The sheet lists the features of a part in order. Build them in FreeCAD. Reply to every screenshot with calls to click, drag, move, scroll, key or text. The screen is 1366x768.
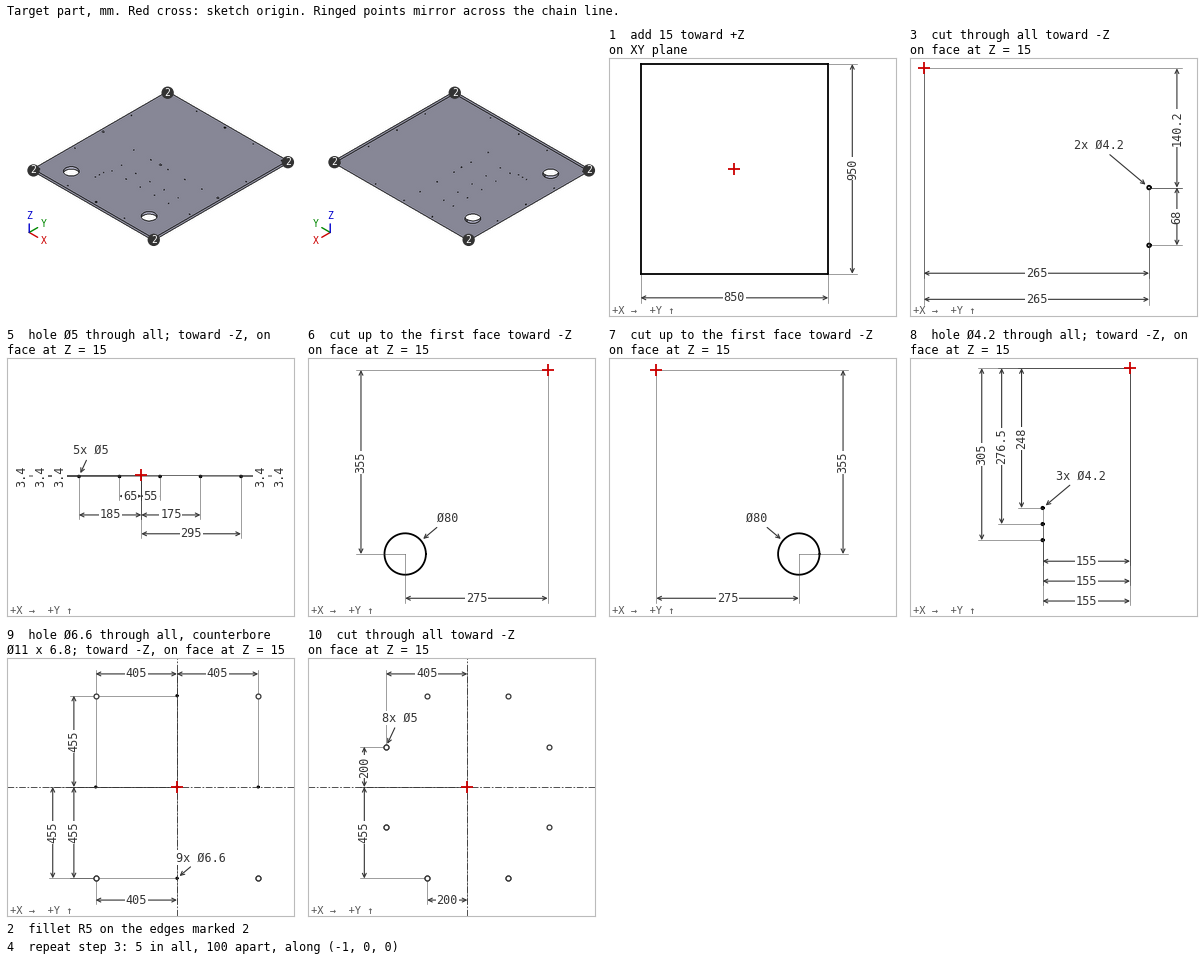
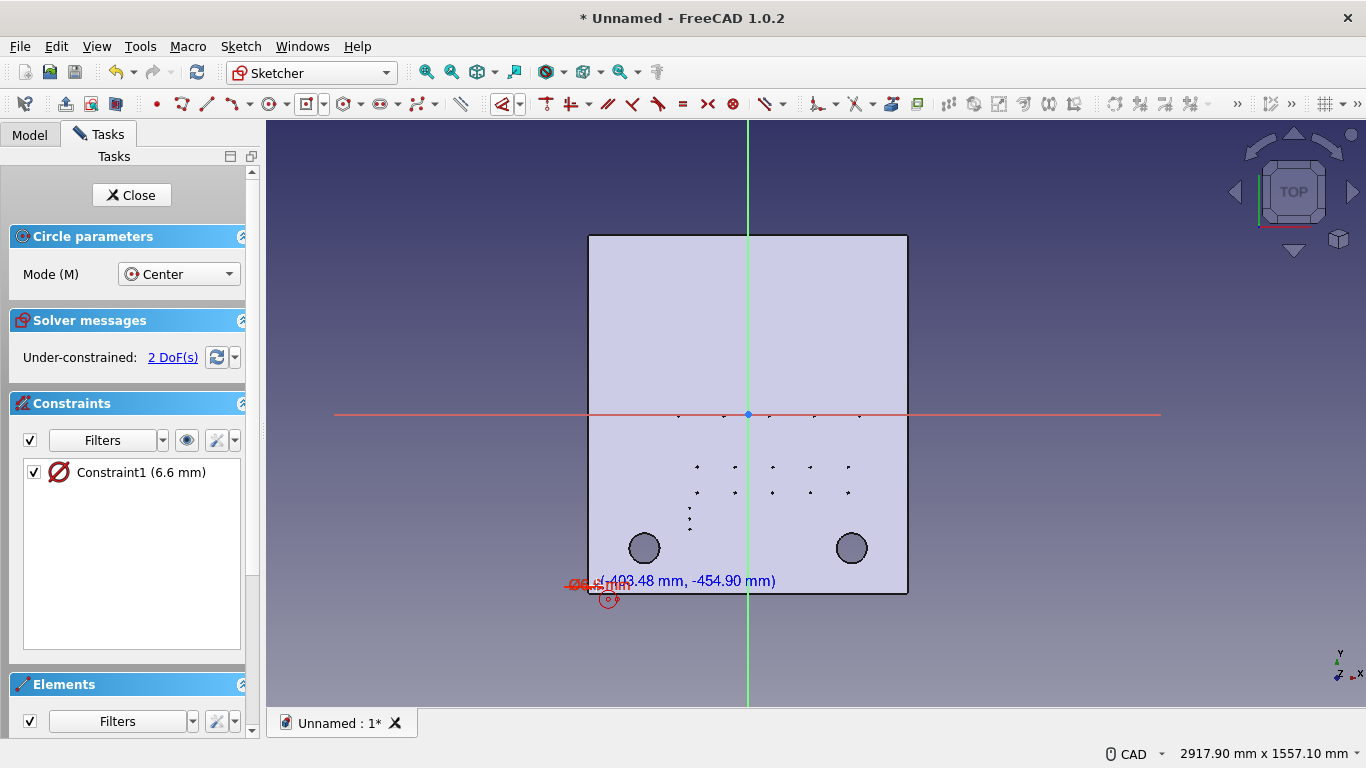
scroll(748, 586, up, 15)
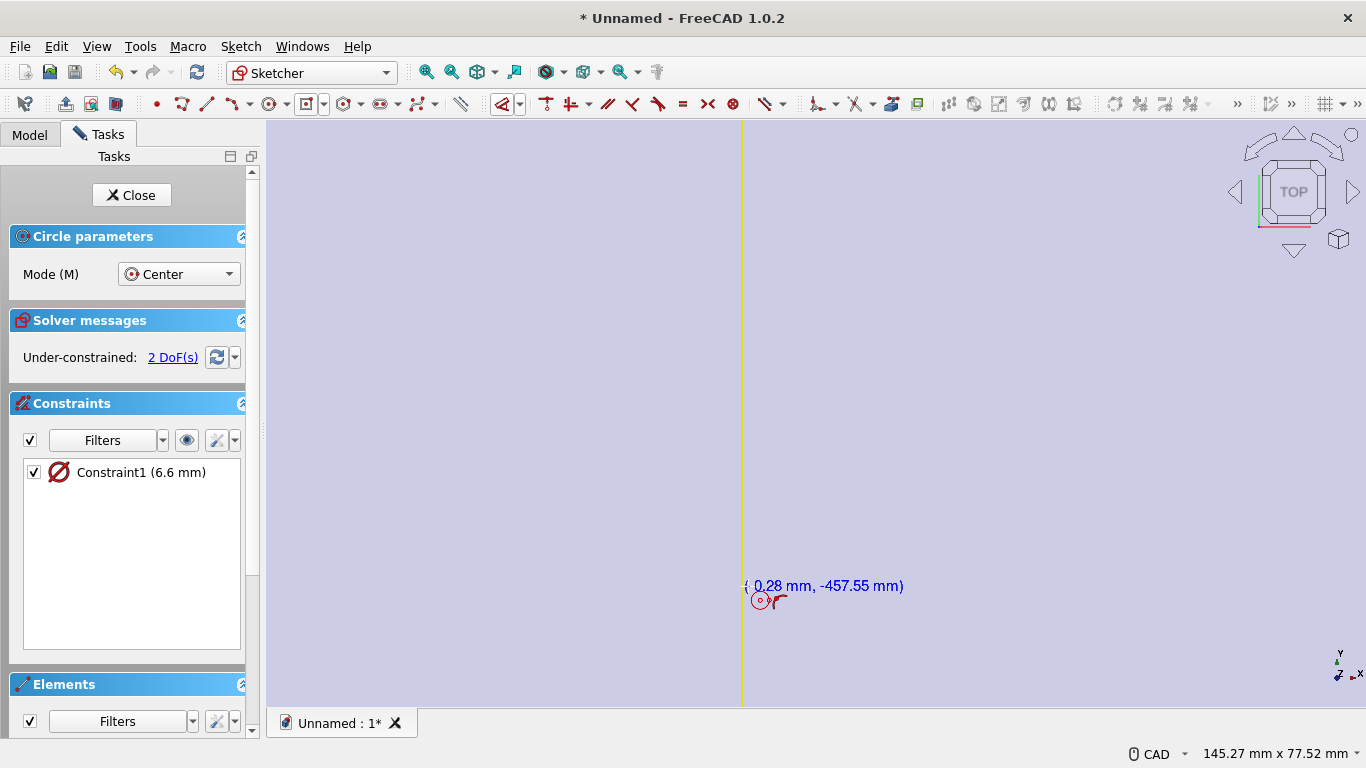
scroll(748, 586, down, 15)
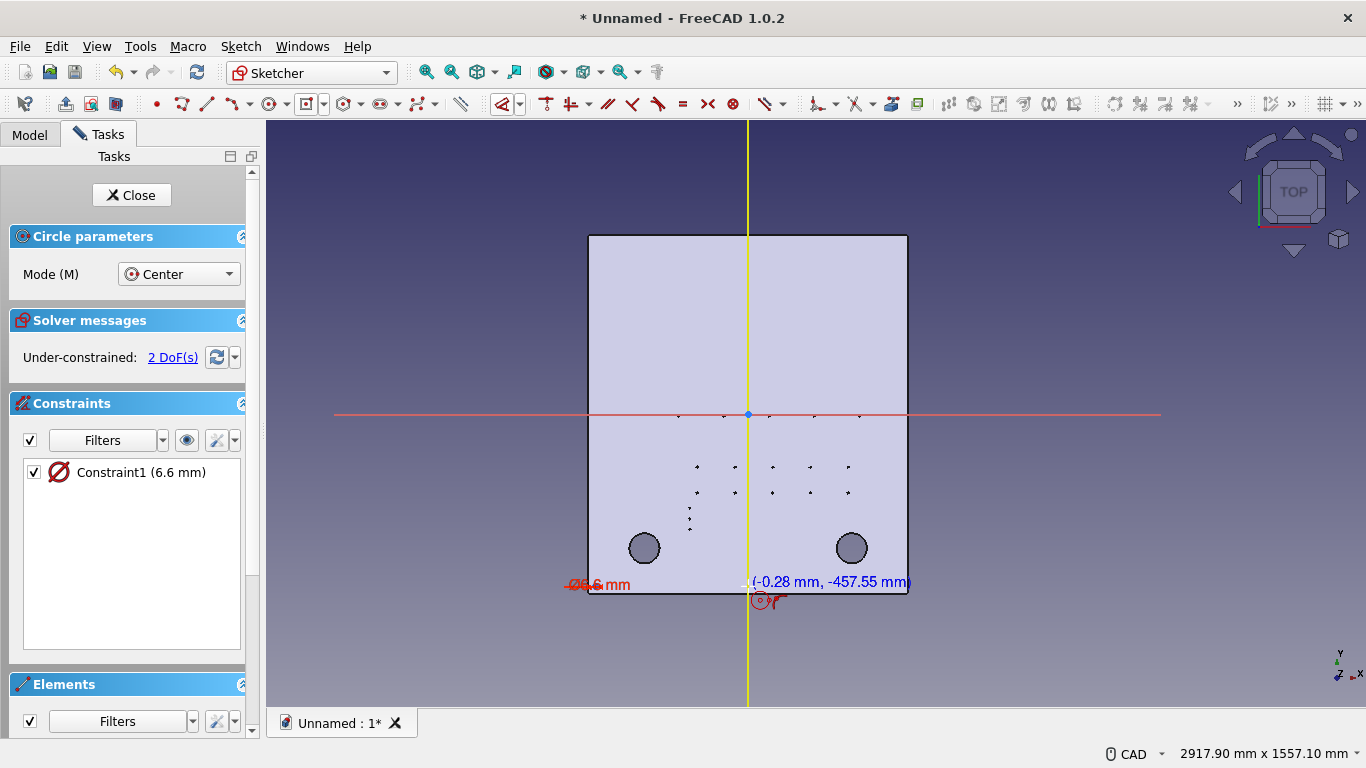
click(748, 586)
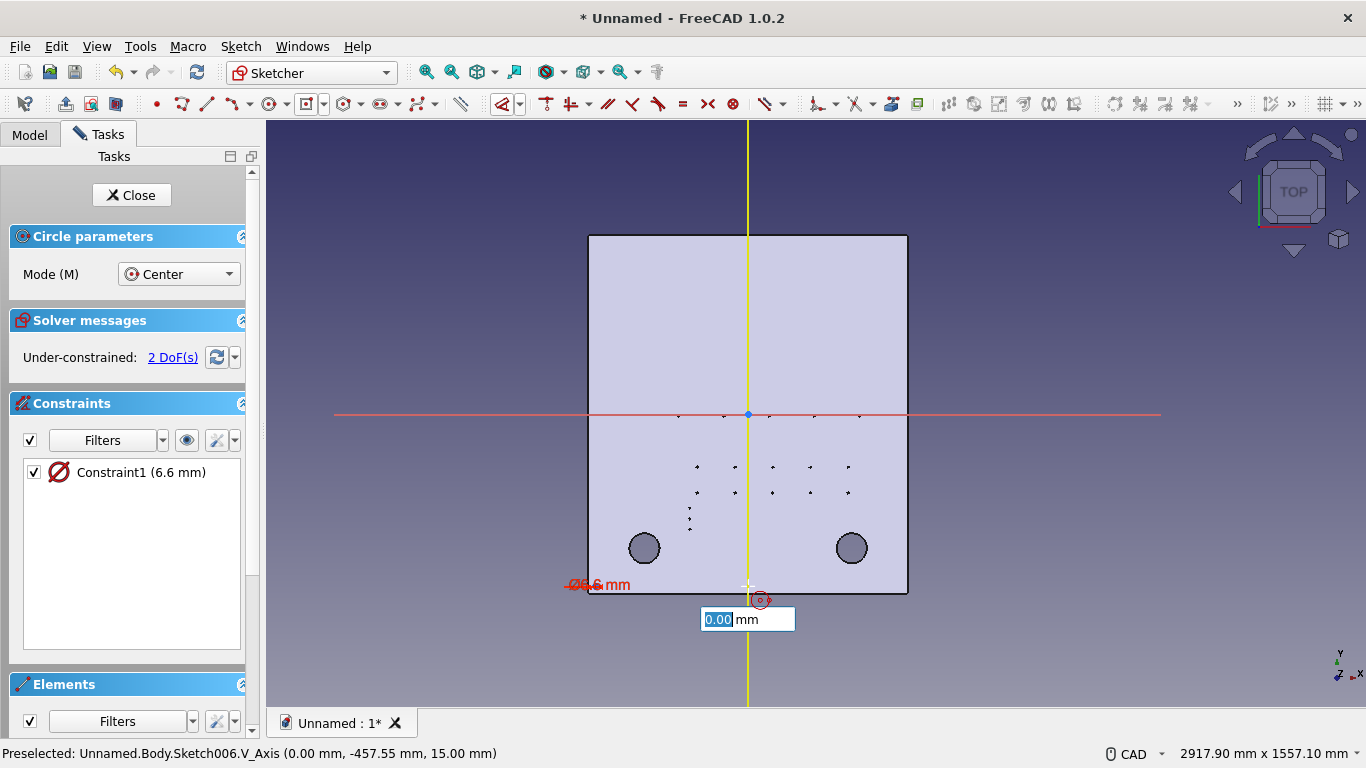
scroll(749, 586, up, 14)
move(747, 567)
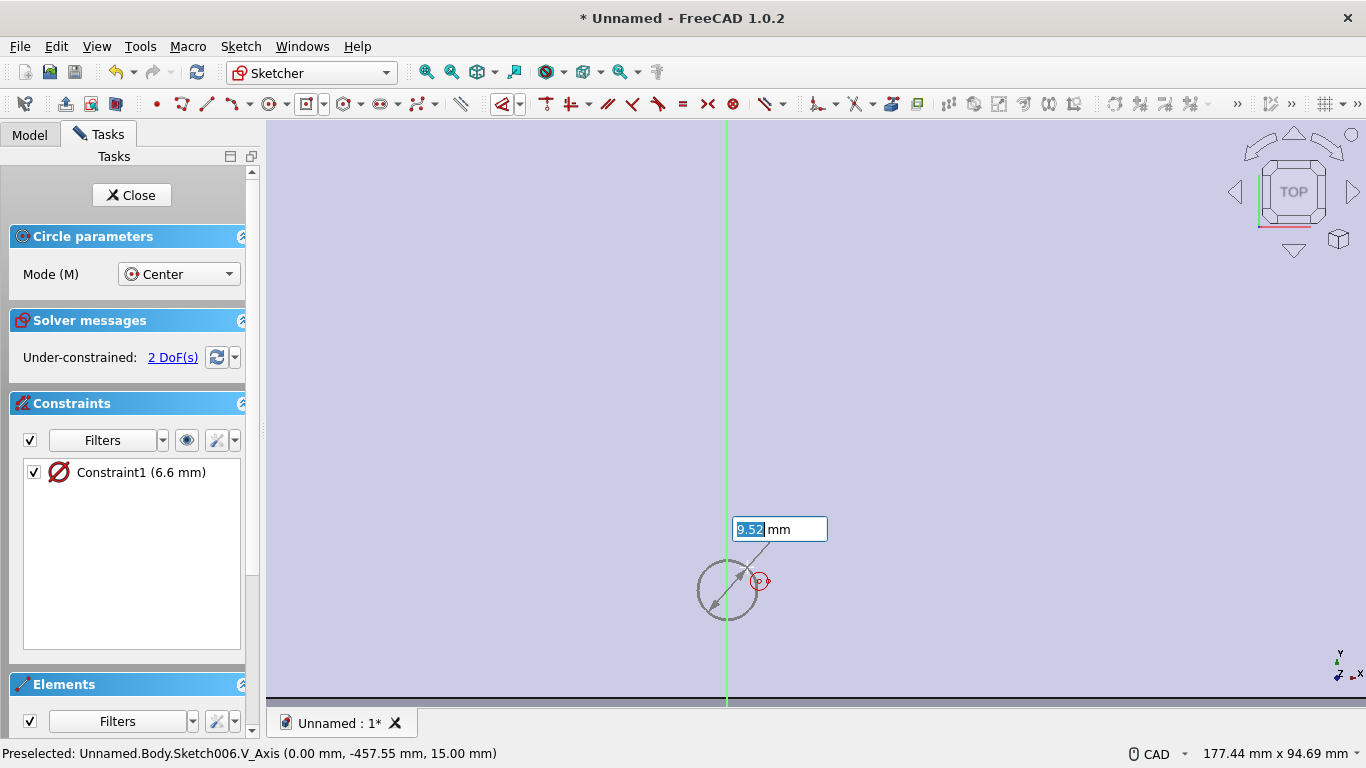
text(6.6)
key(Return)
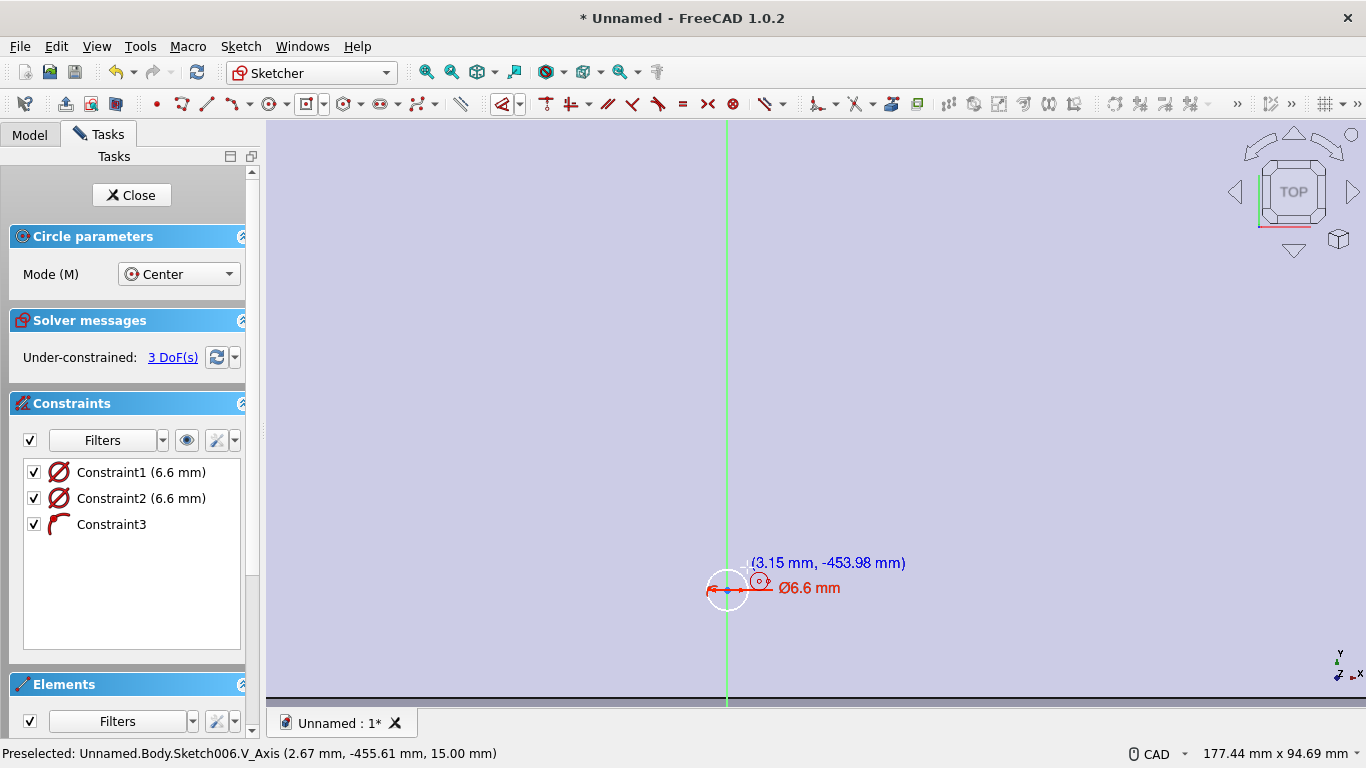
scroll(749, 586, down, 14)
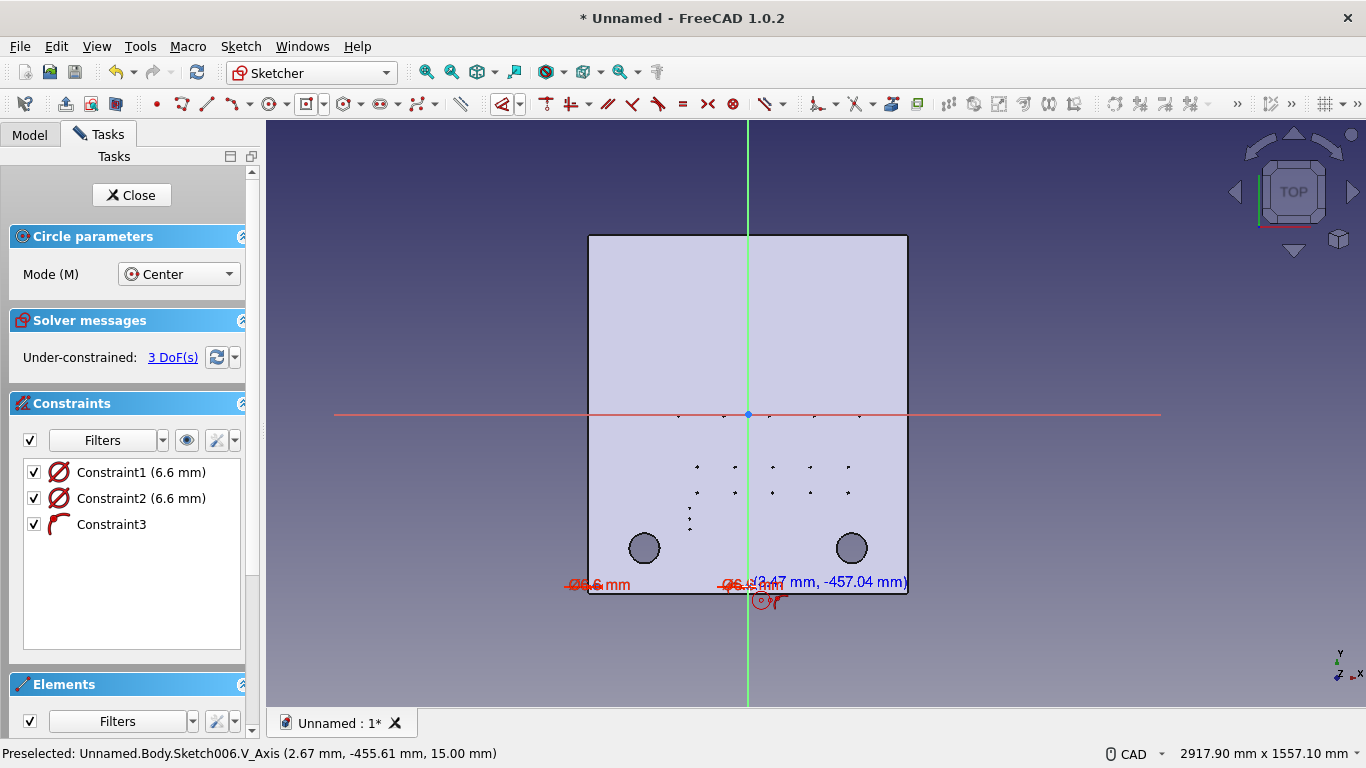
scroll(901, 586, up, 15)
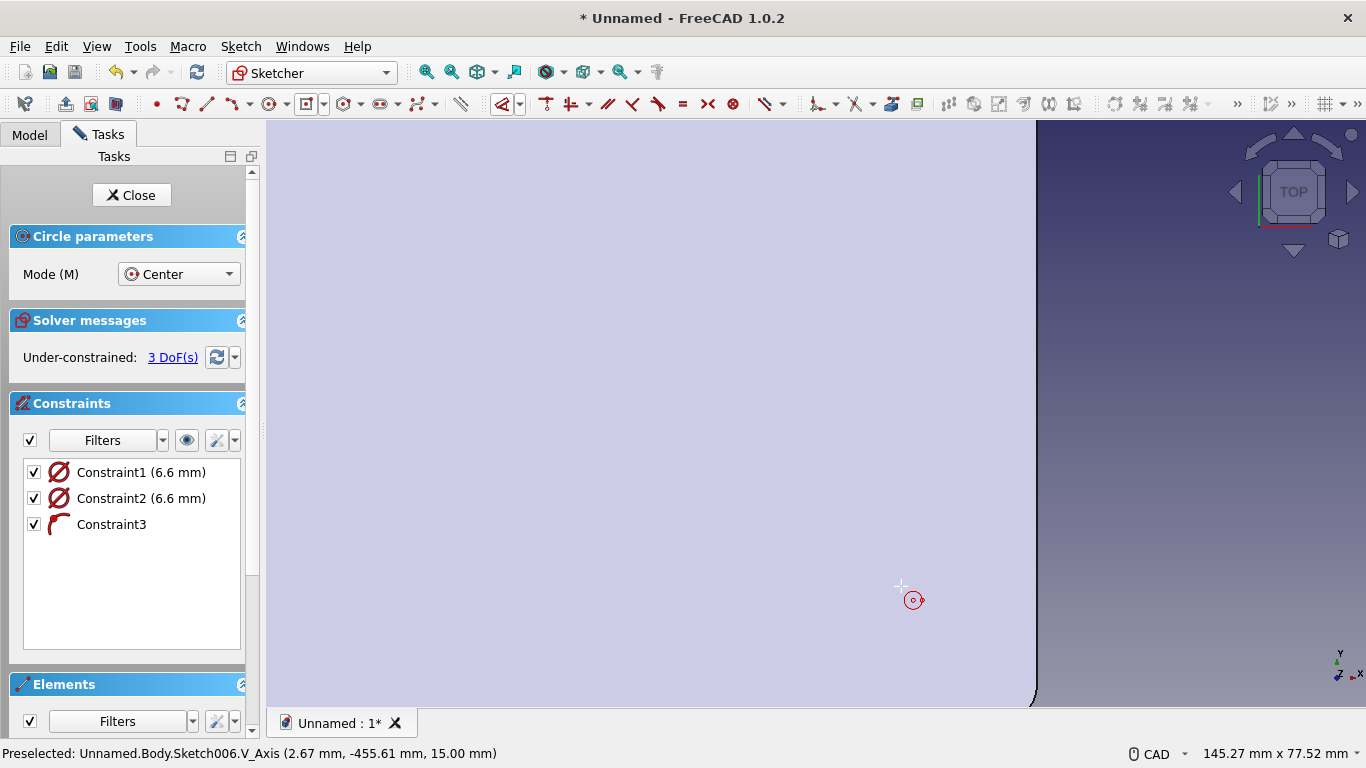
scroll(901, 586, down, 15)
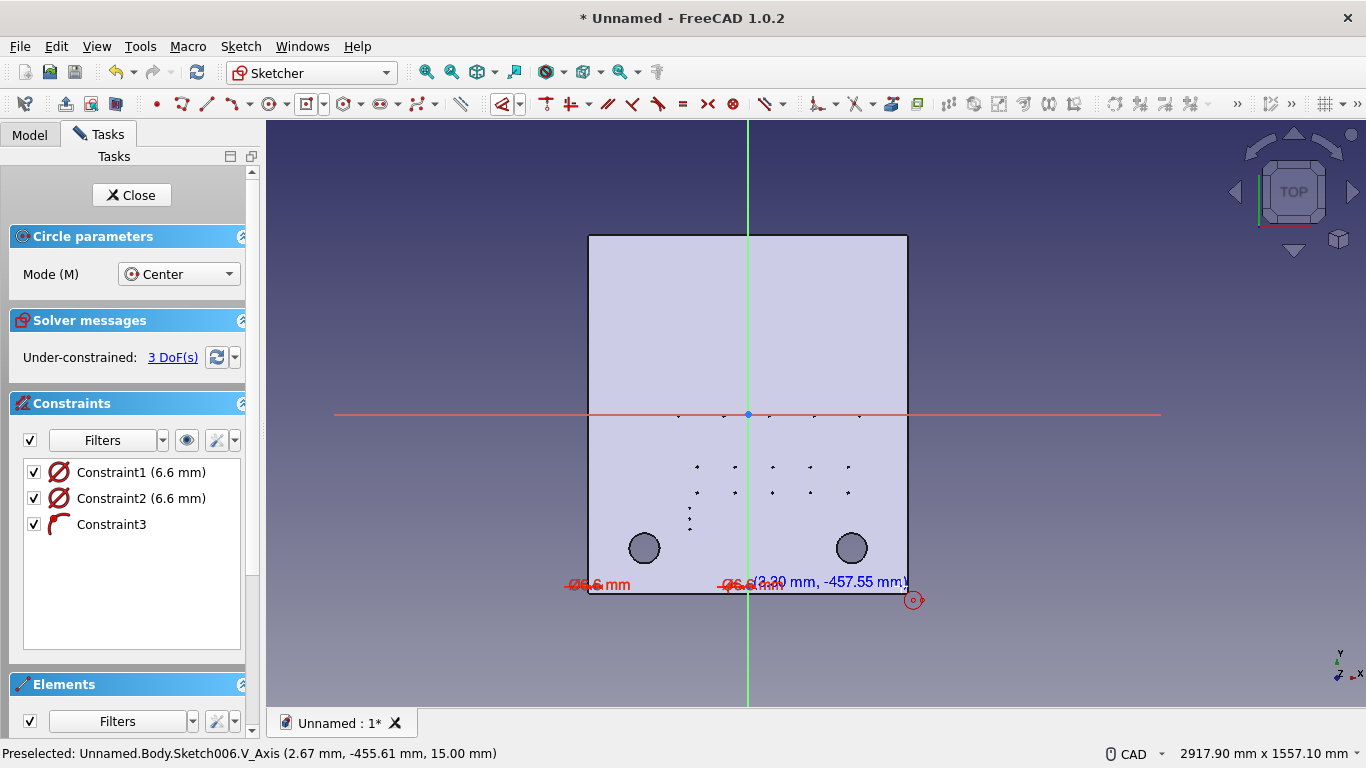
click(901, 586)
move(902, 585)